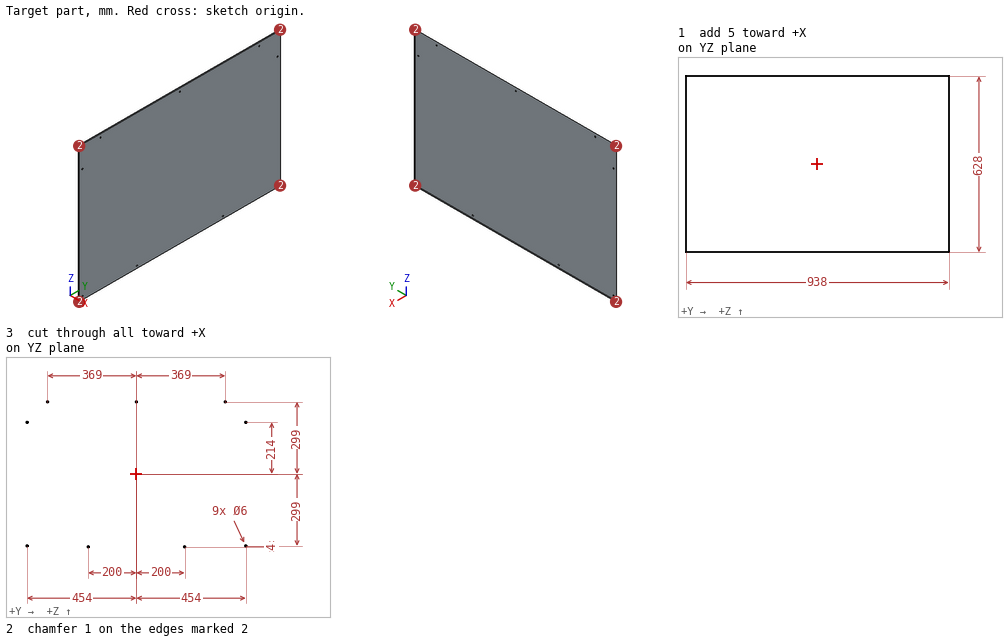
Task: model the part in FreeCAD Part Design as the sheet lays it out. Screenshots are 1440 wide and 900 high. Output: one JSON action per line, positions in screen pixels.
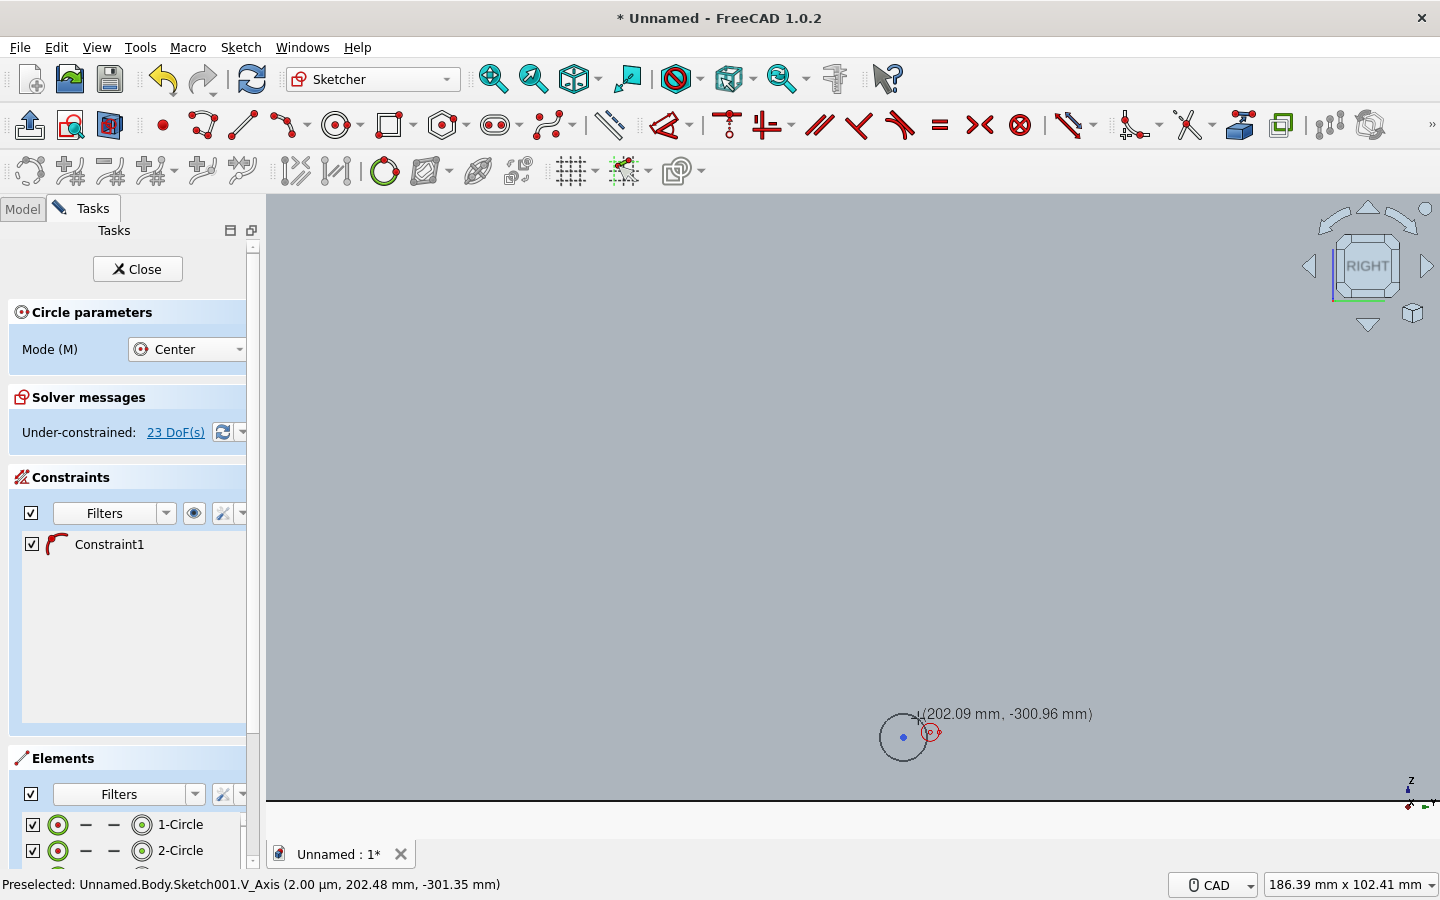
{"action": "scroll", "coordinate": [926, 726], "scroll_direction": "down", "scroll_amount": 11}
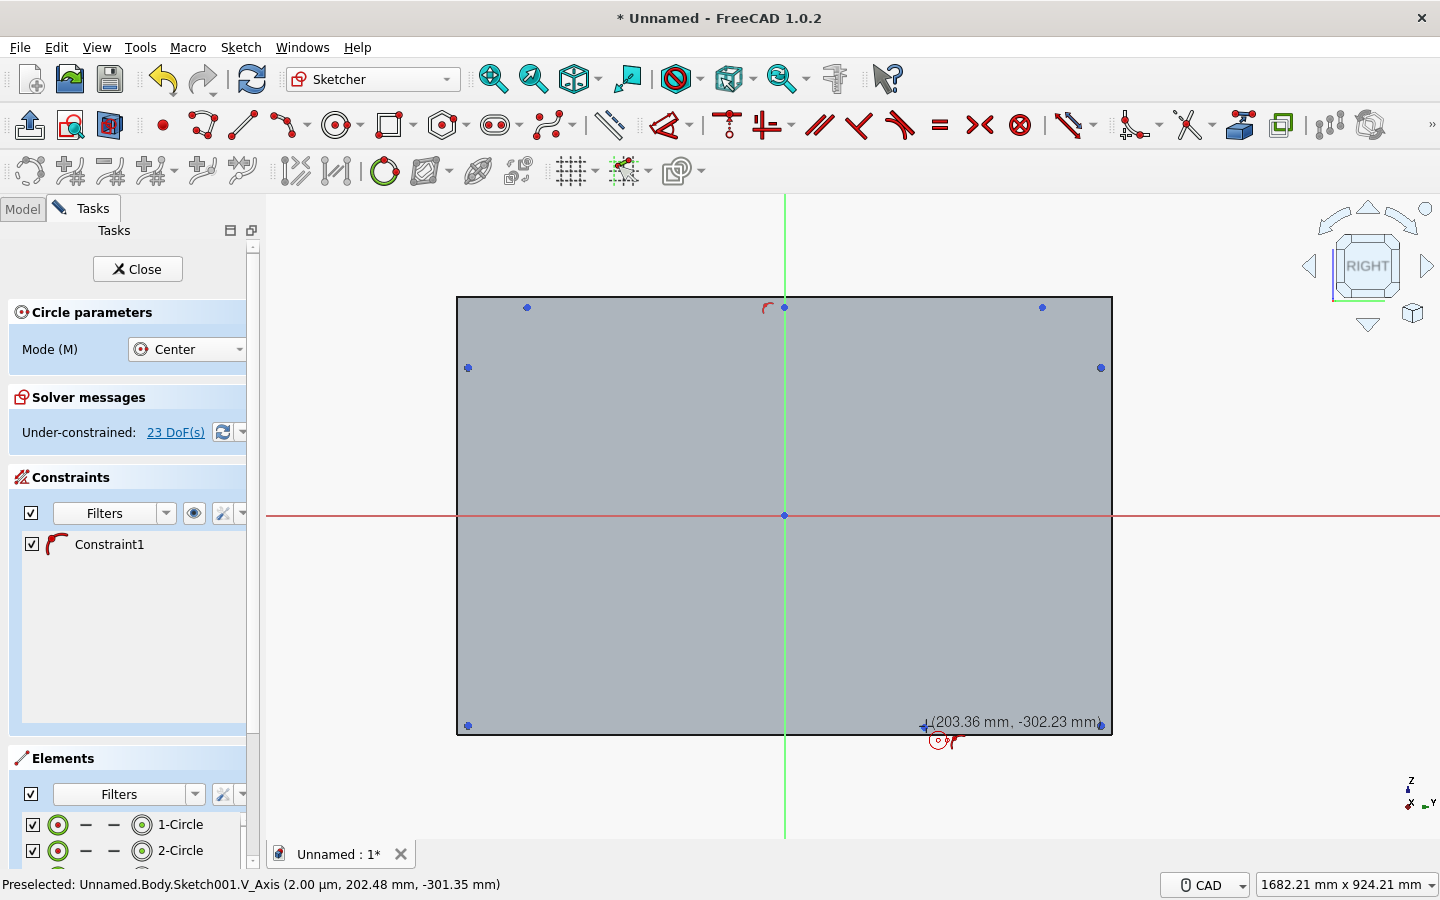
{"action": "scroll", "coordinate": [645, 727], "scroll_direction": "up", "scroll_amount": 12}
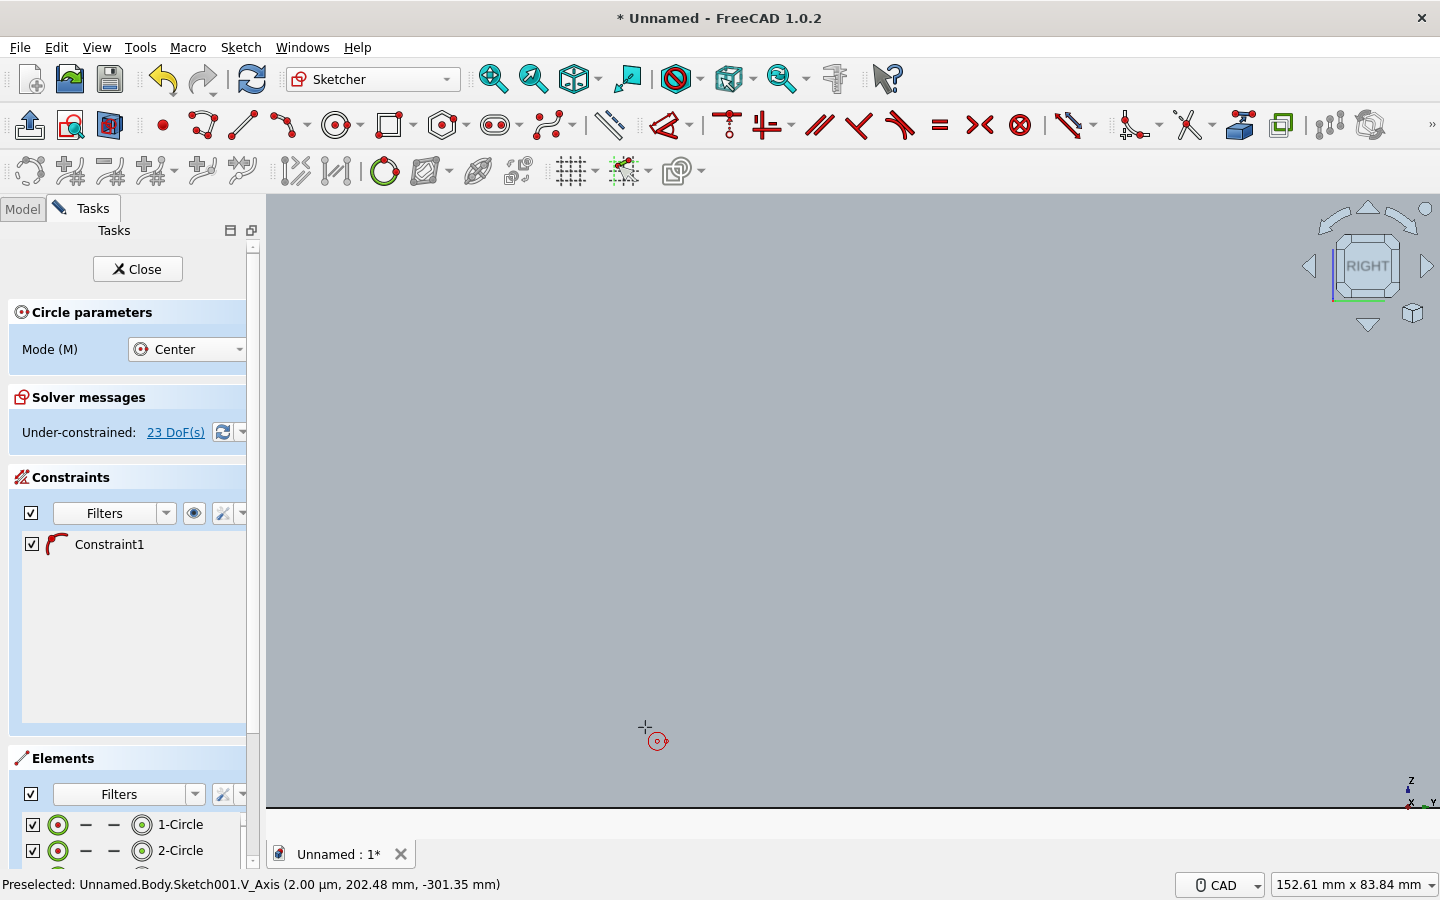
{"action": "scroll", "coordinate": [645, 727], "scroll_direction": "down", "scroll_amount": 12}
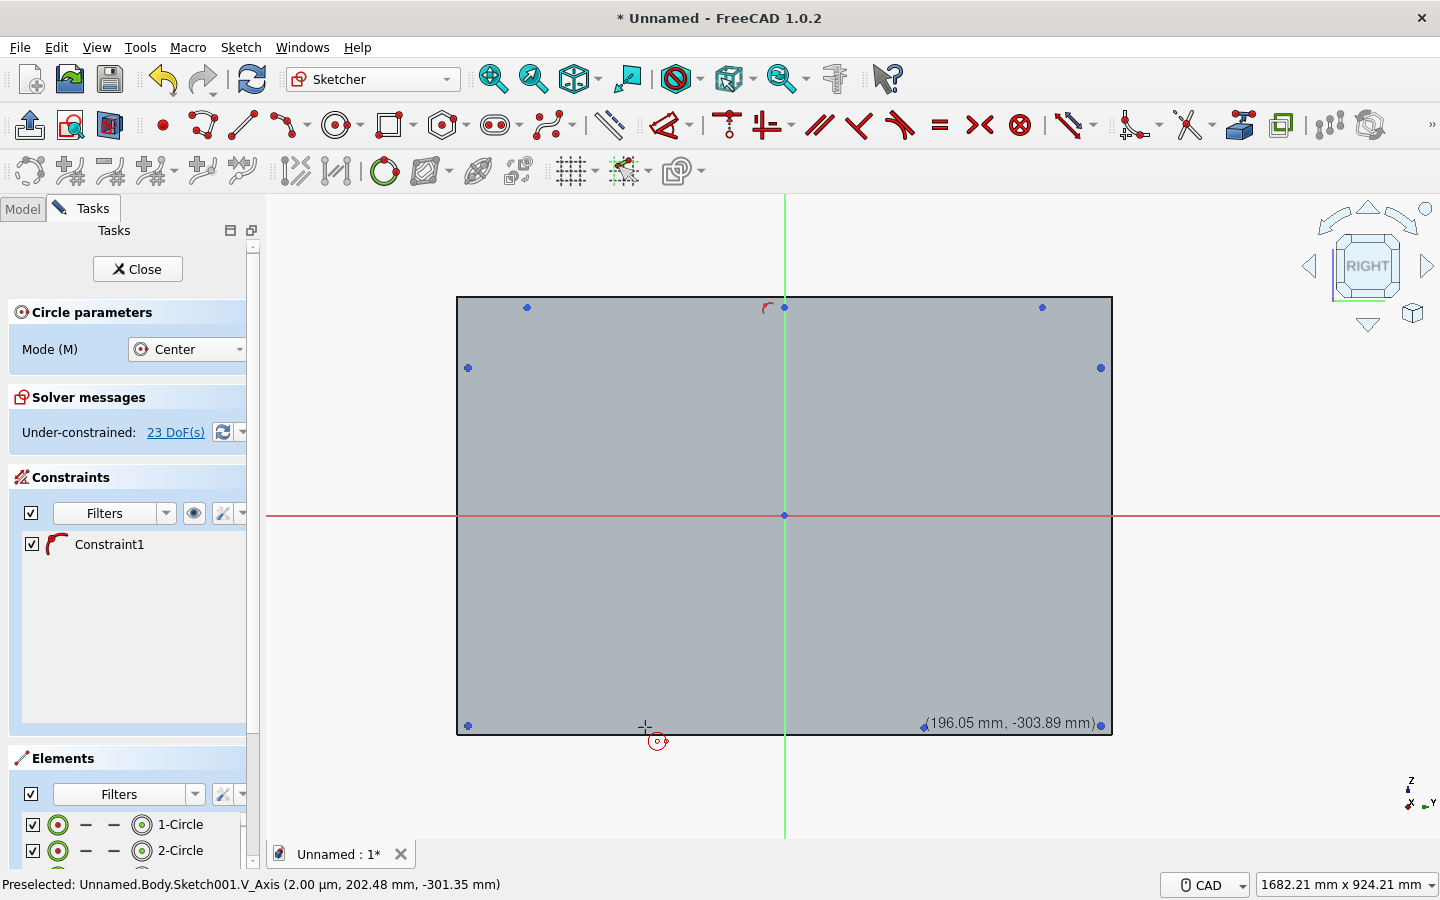
{"action": "left_click", "coordinate": [645, 727]}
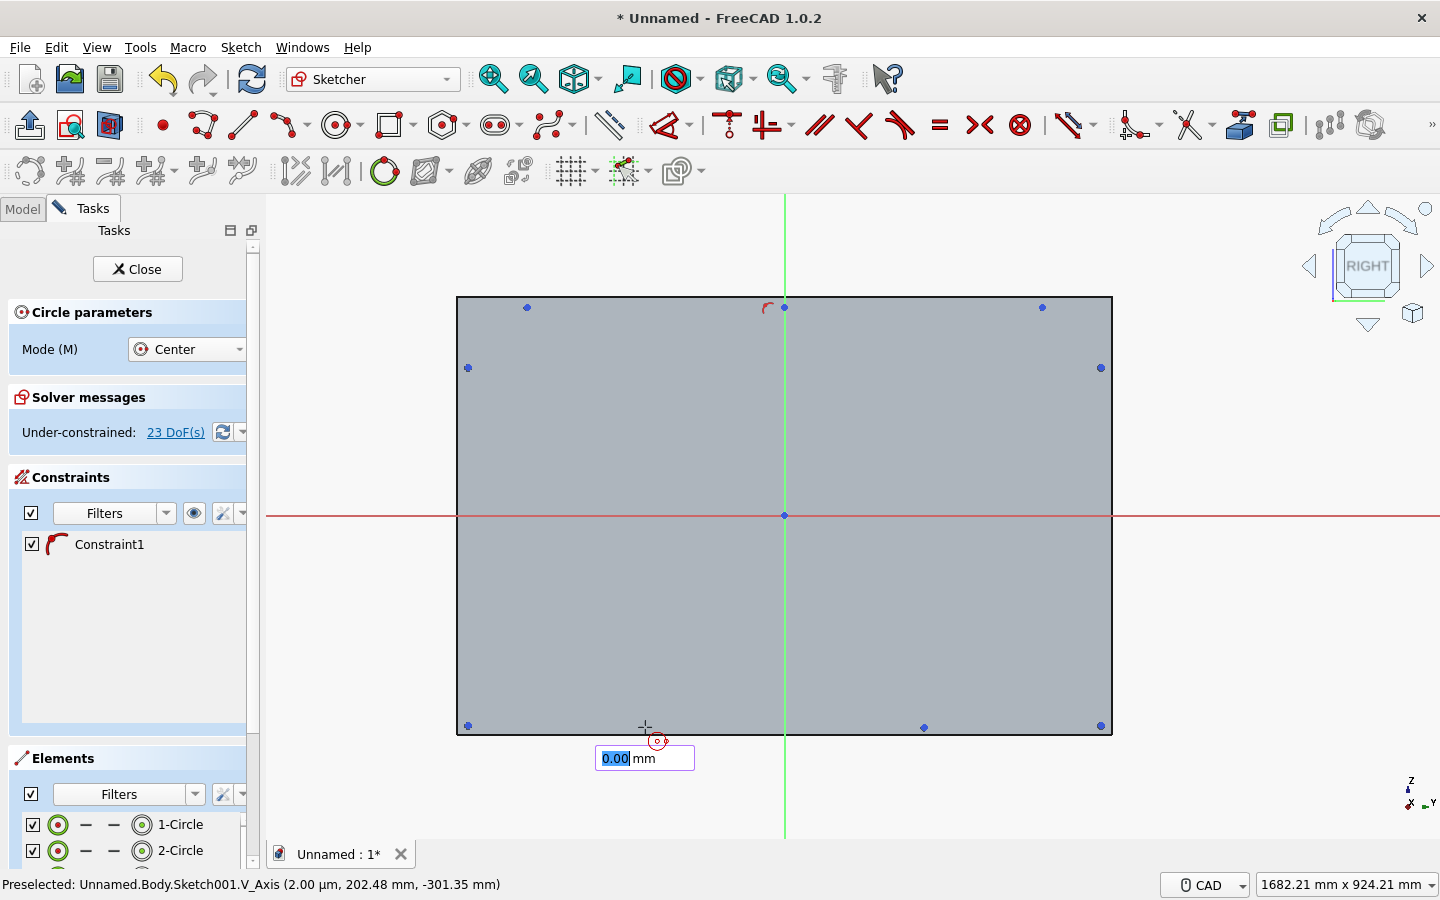
{"action": "scroll", "coordinate": [646, 726], "scroll_direction": "up", "scroll_amount": 11}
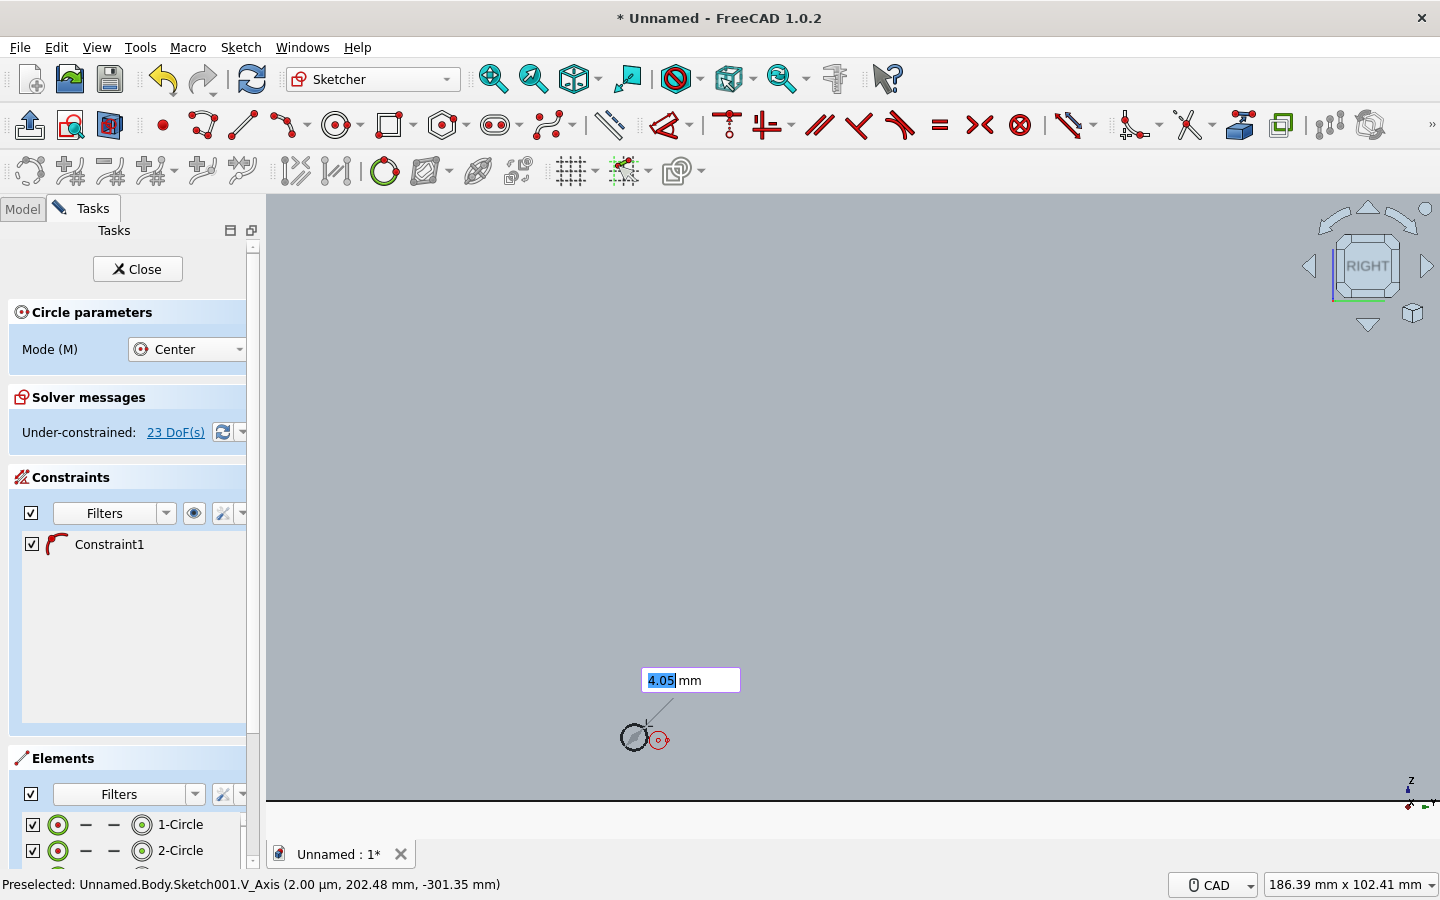
{"action": "left_click", "coordinate": [648, 718]}
{"action": "key", "text": "Escape"}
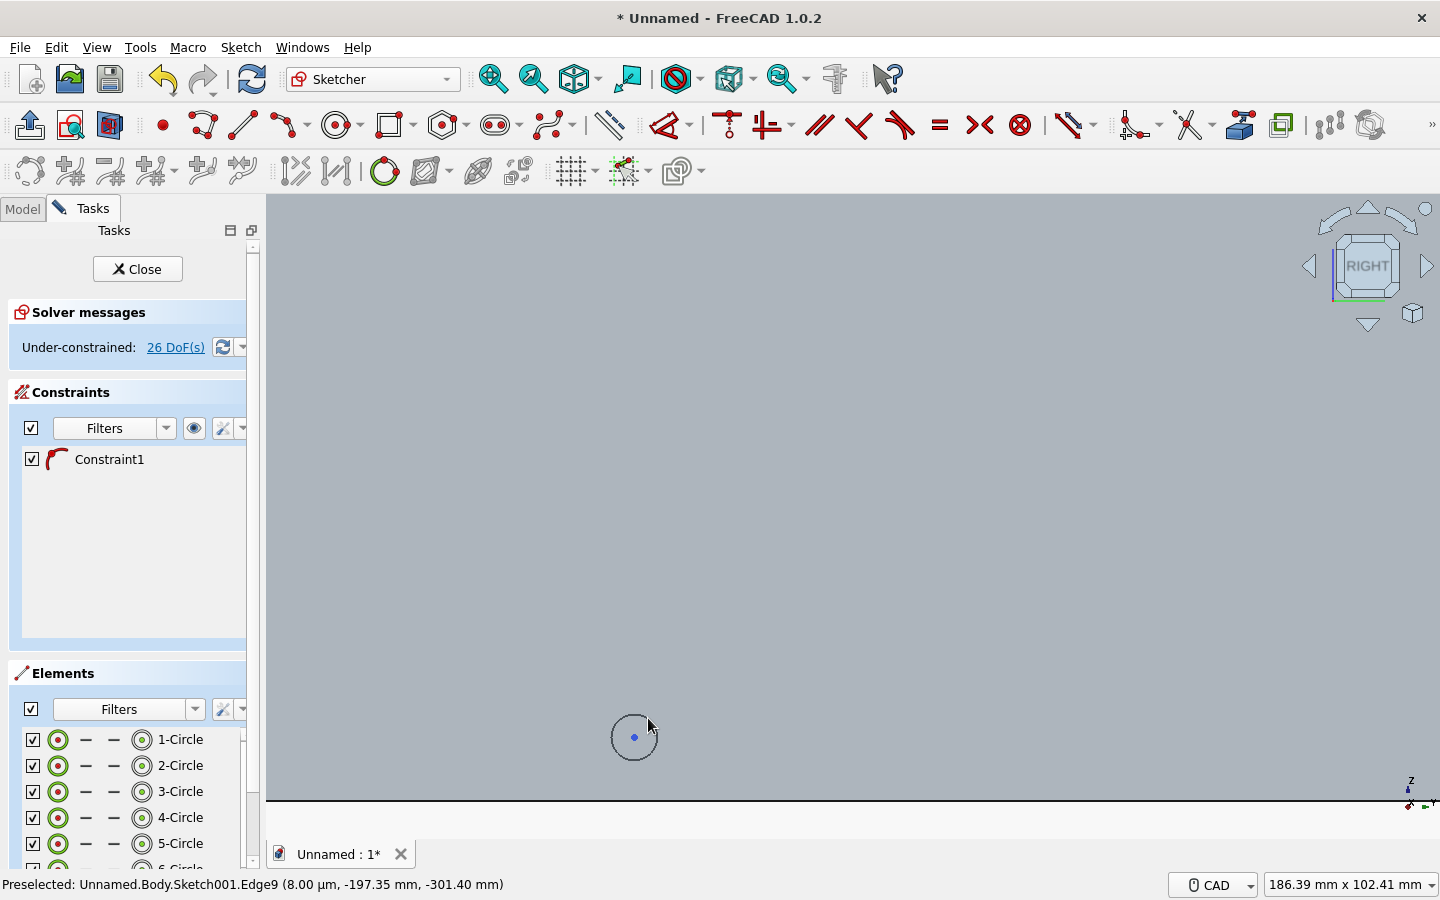
{"action": "scroll", "coordinate": [646, 726], "scroll_direction": "down", "scroll_amount": 11}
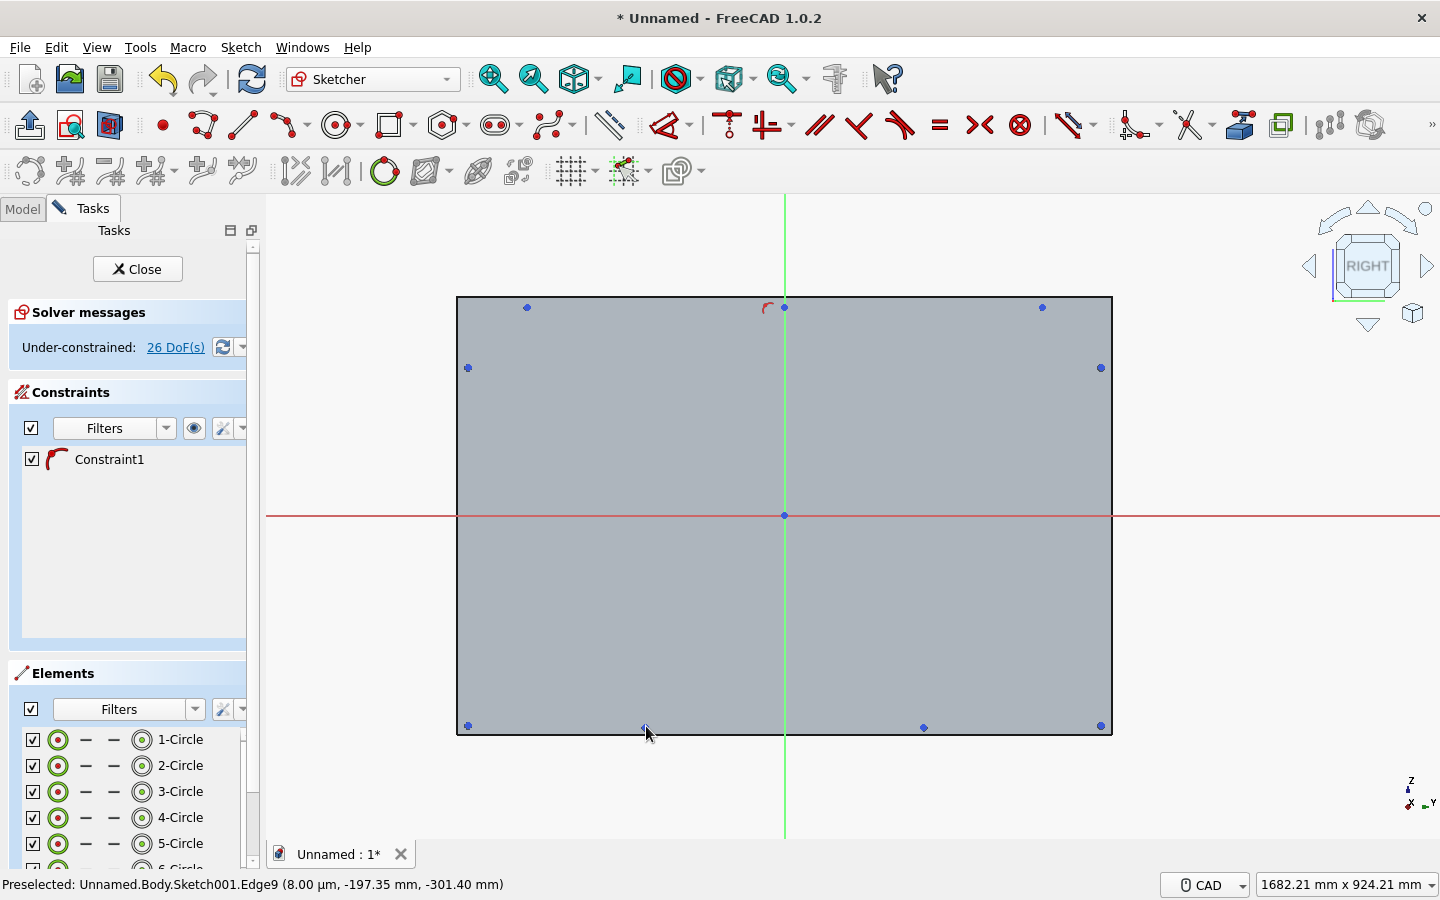
{"action": "scroll", "coordinate": [1103, 724], "scroll_direction": "up", "scroll_amount": 8}